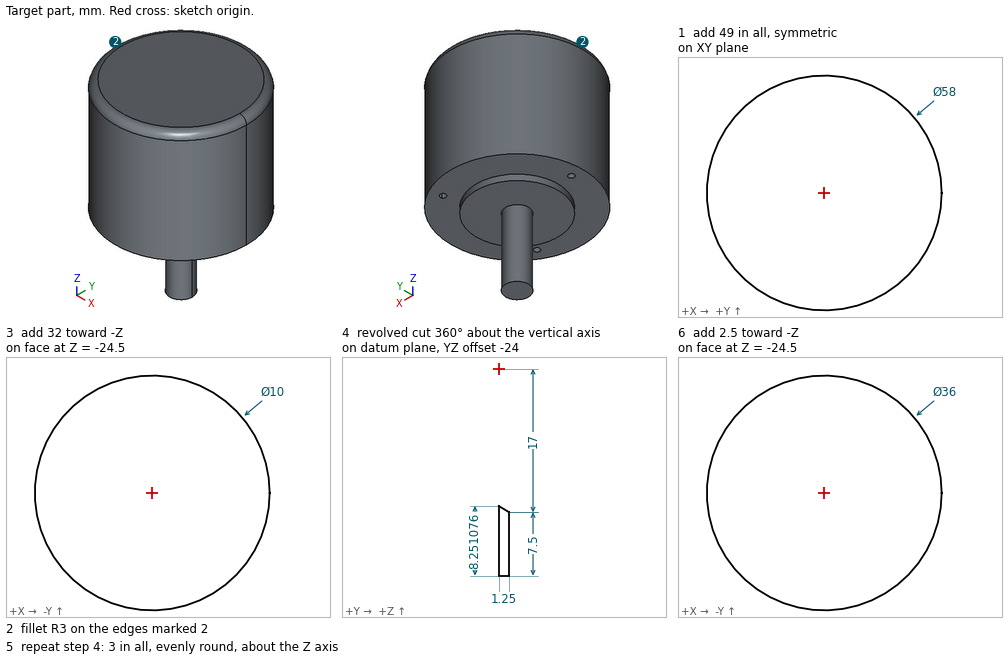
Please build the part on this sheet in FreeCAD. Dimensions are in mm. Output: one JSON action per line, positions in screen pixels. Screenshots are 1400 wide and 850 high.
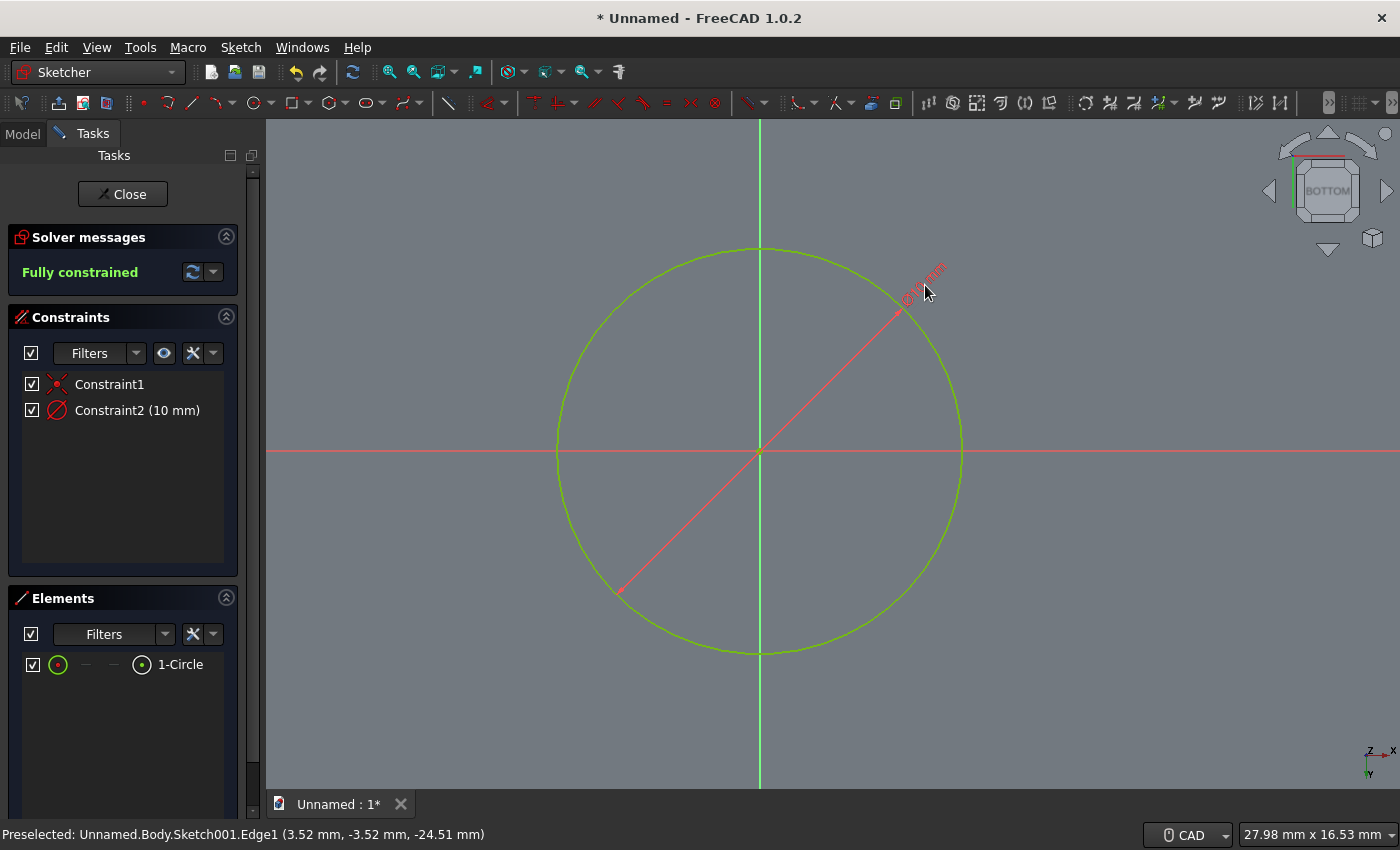
{"action": "left_click", "coordinate": [123, 194]}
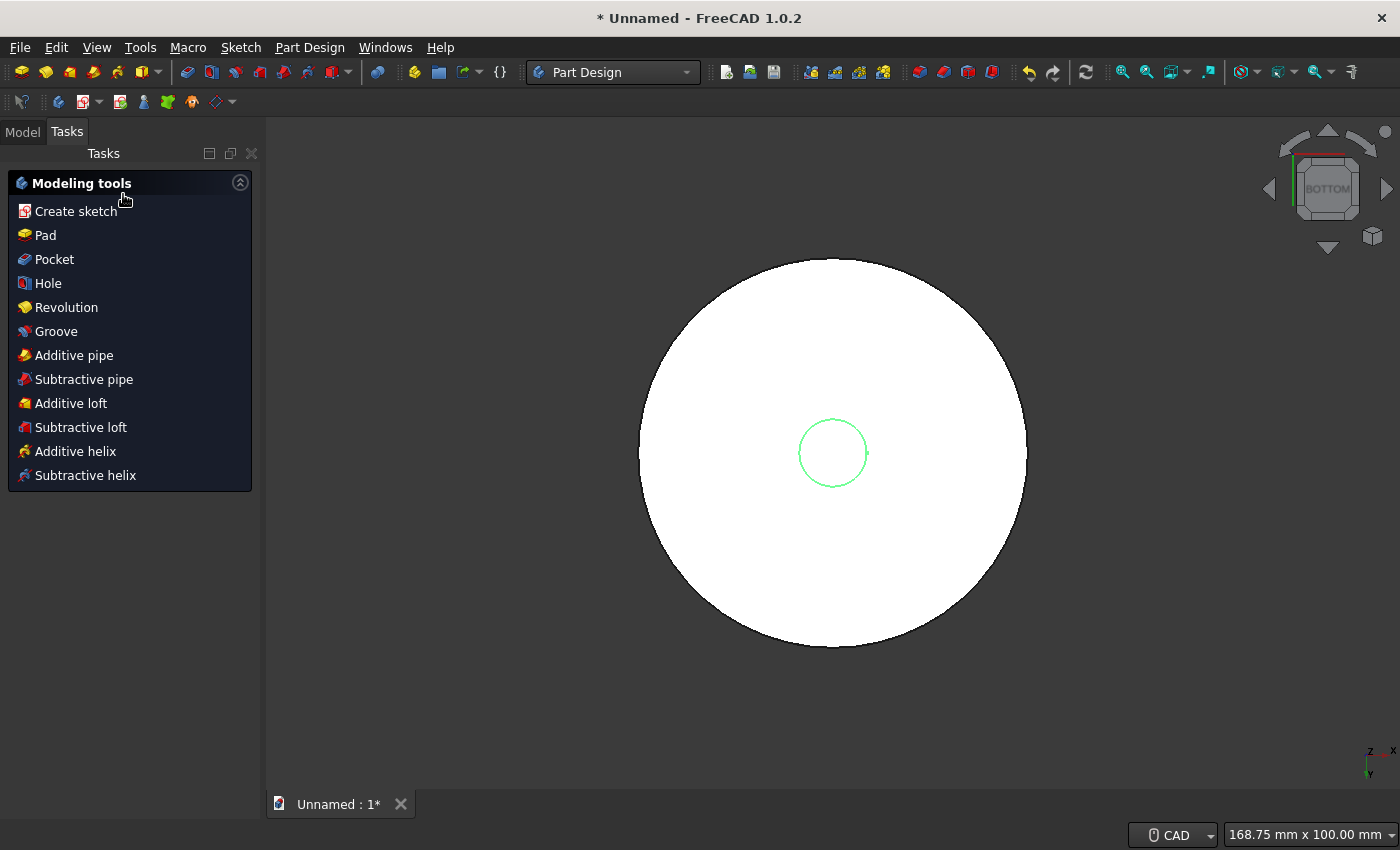
{"action": "left_click", "coordinate": [22, 72]}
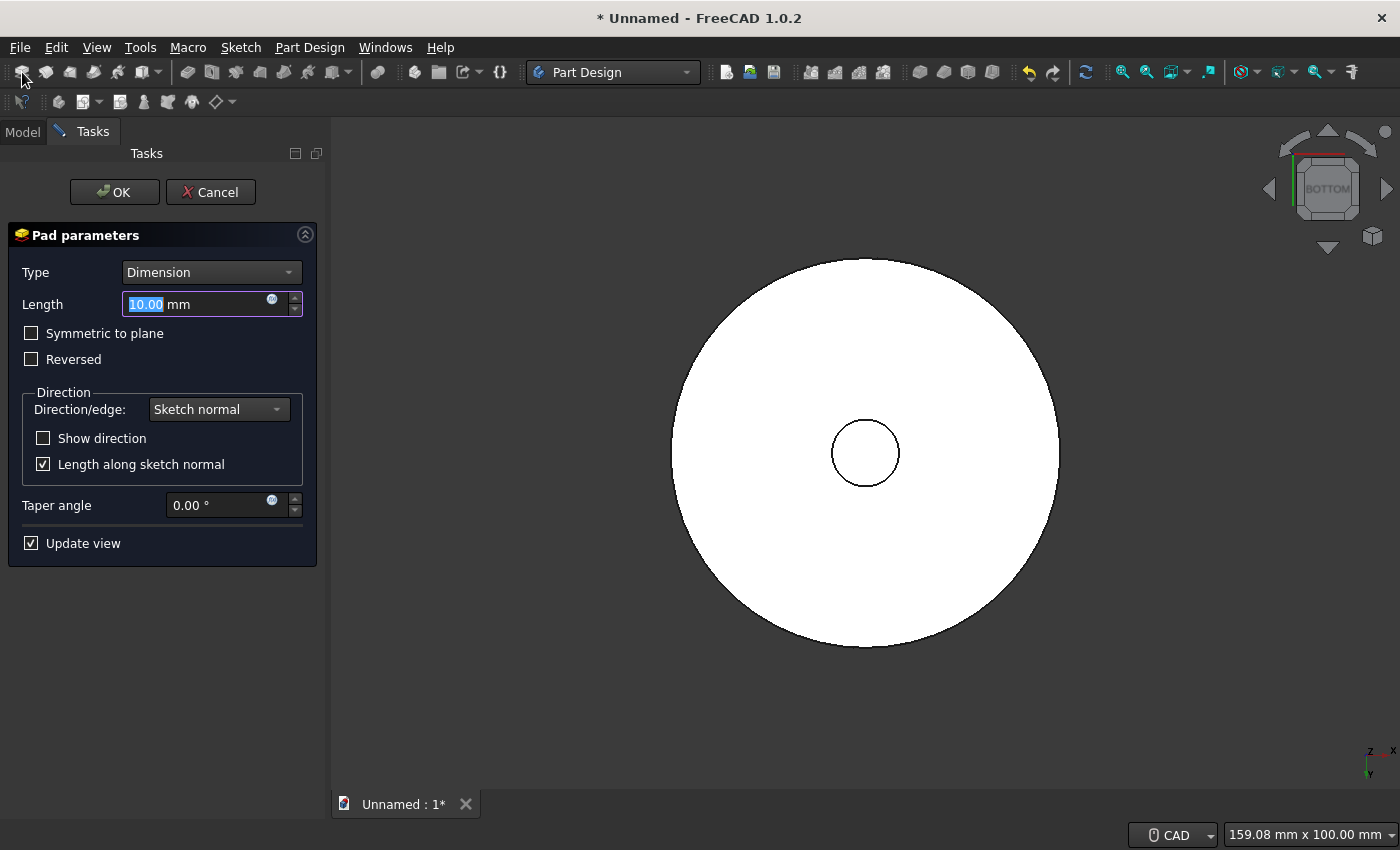
{"action": "type", "text": "32"}
{"action": "key", "text": "Tab"}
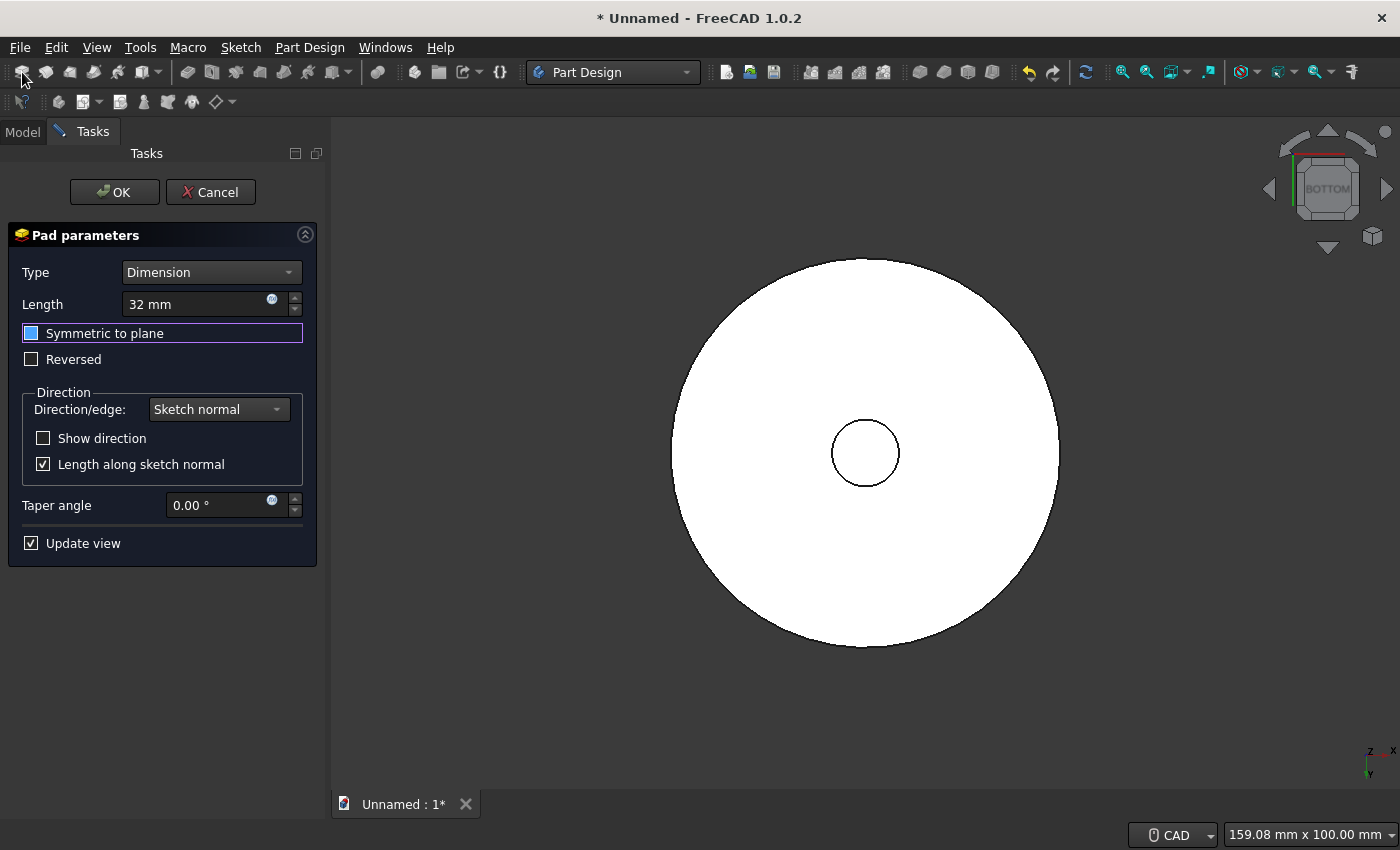
{"action": "left_click", "coordinate": [115, 192]}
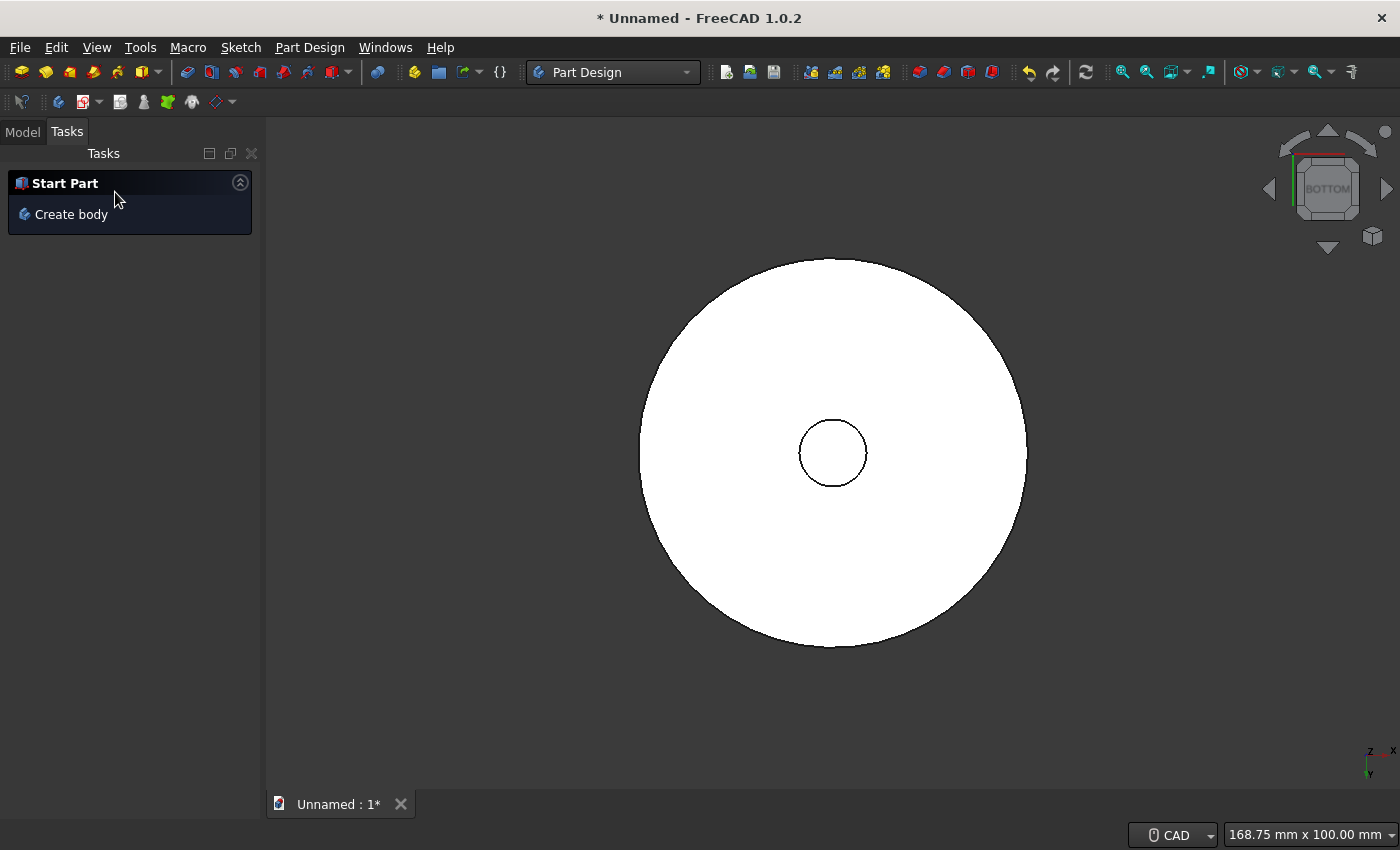
{"action": "left_click", "coordinate": [23, 131]}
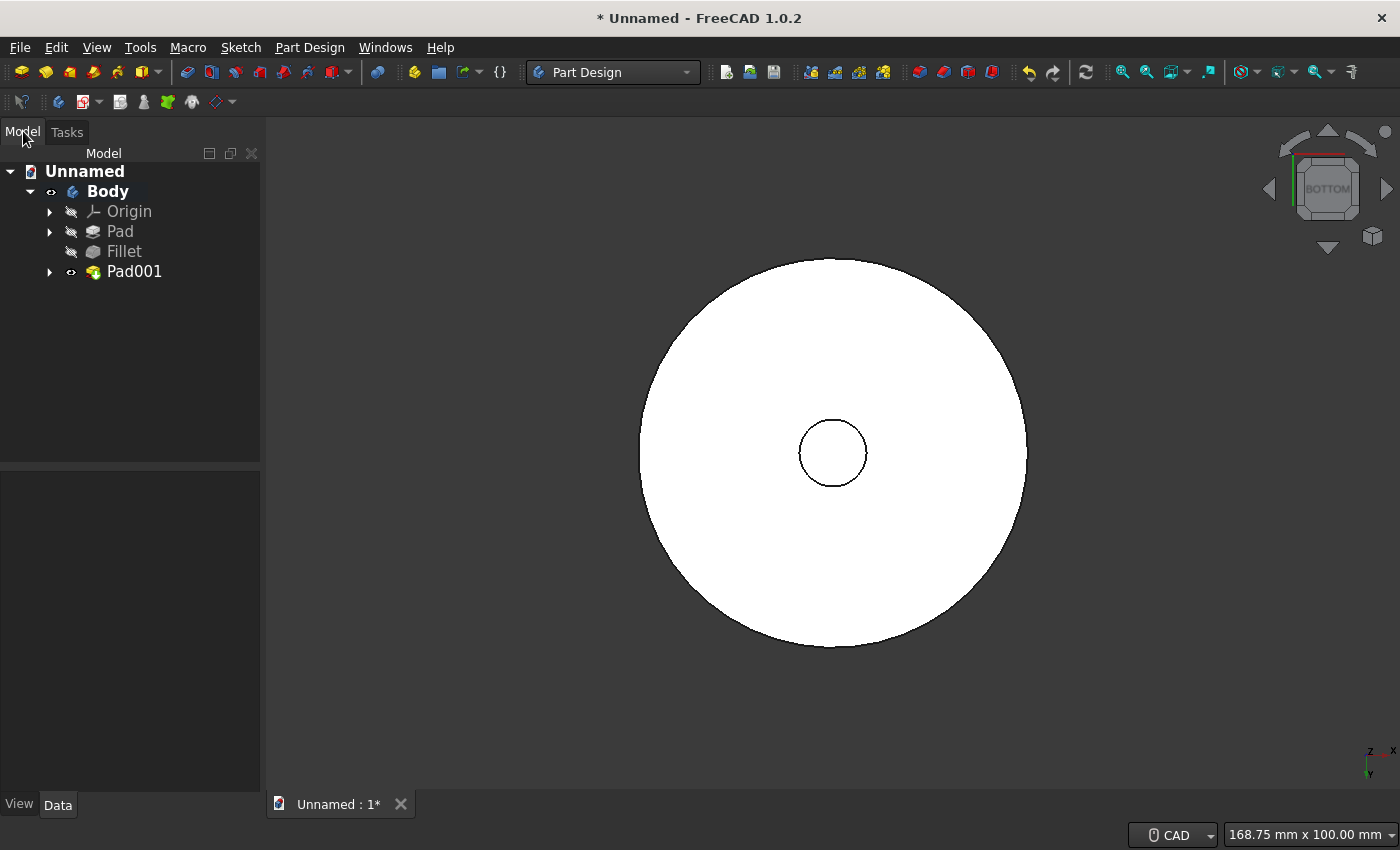
{"action": "left_click", "coordinate": [50, 212]}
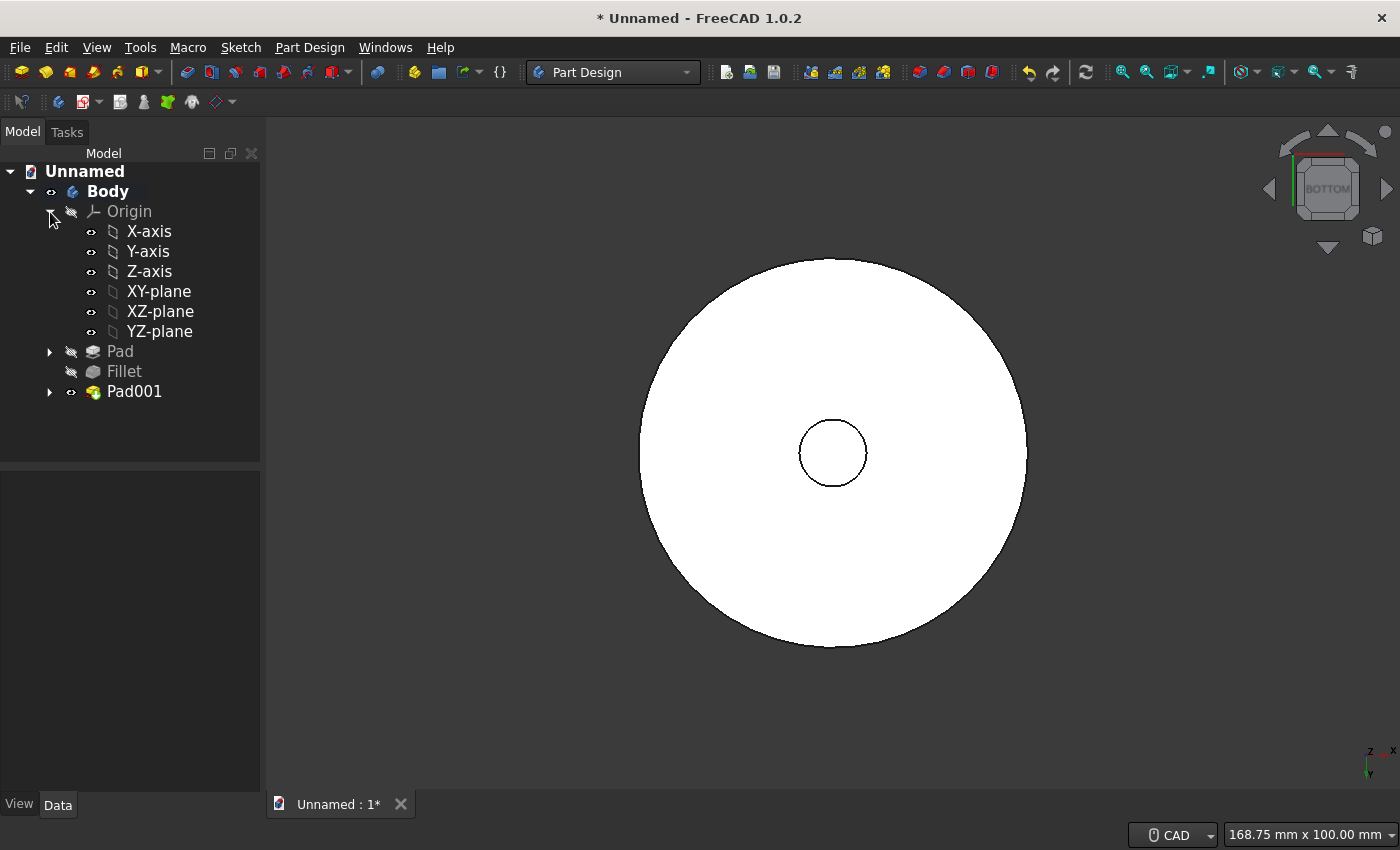
{"action": "left_click", "coordinate": [136, 332]}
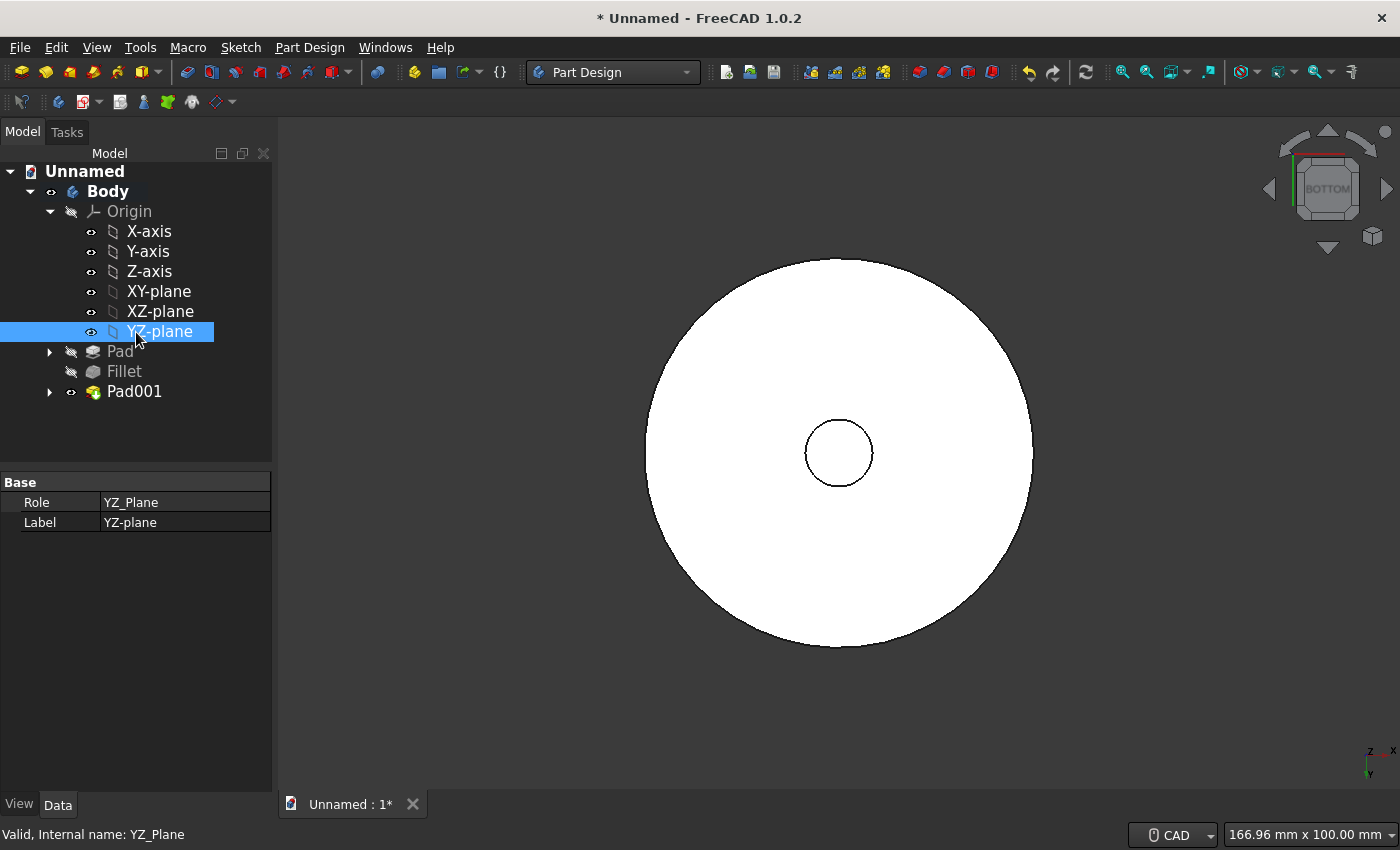
{"action": "left_click", "coordinate": [216, 102]}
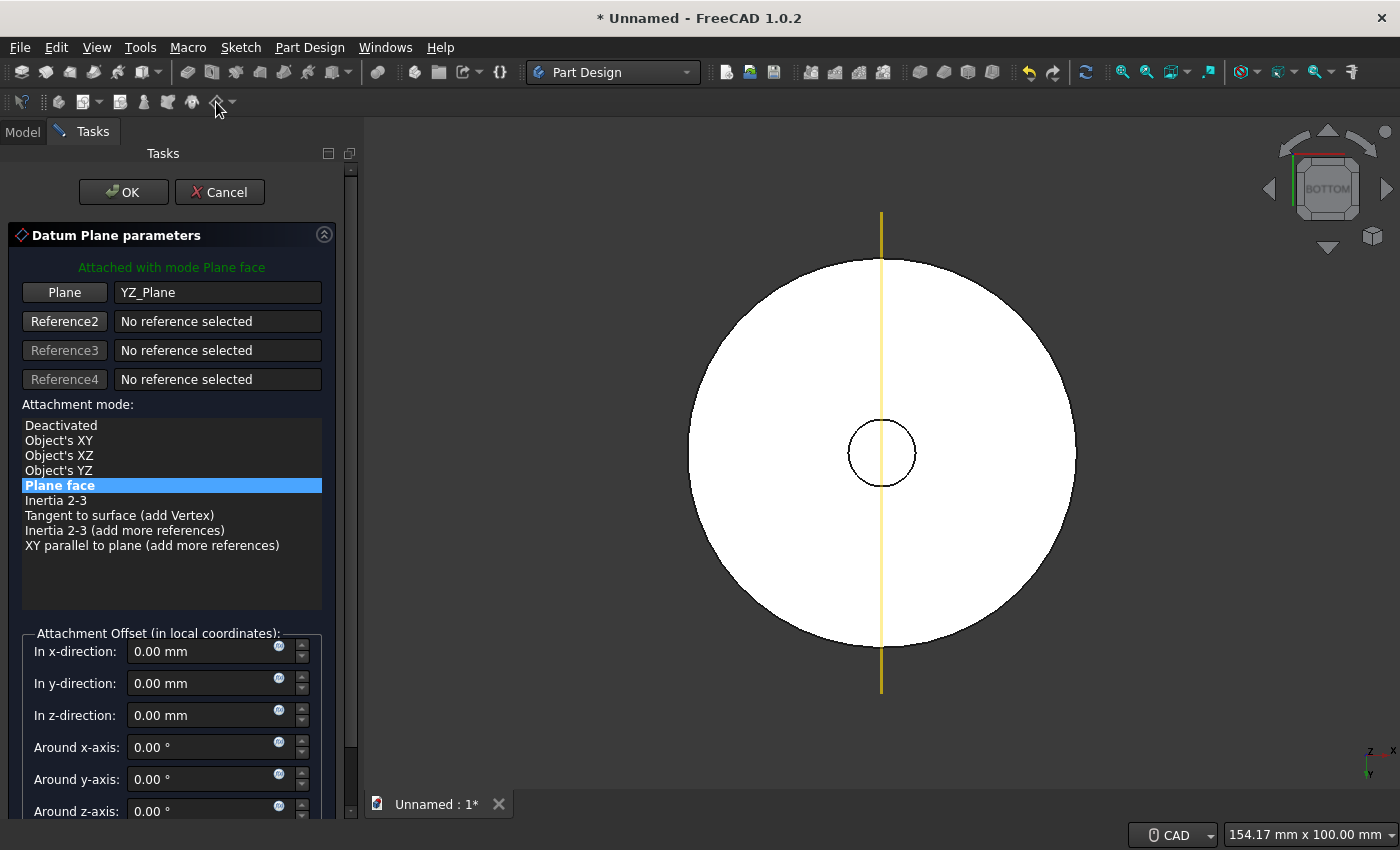
{"action": "triple_click", "coordinate": [210, 715]}